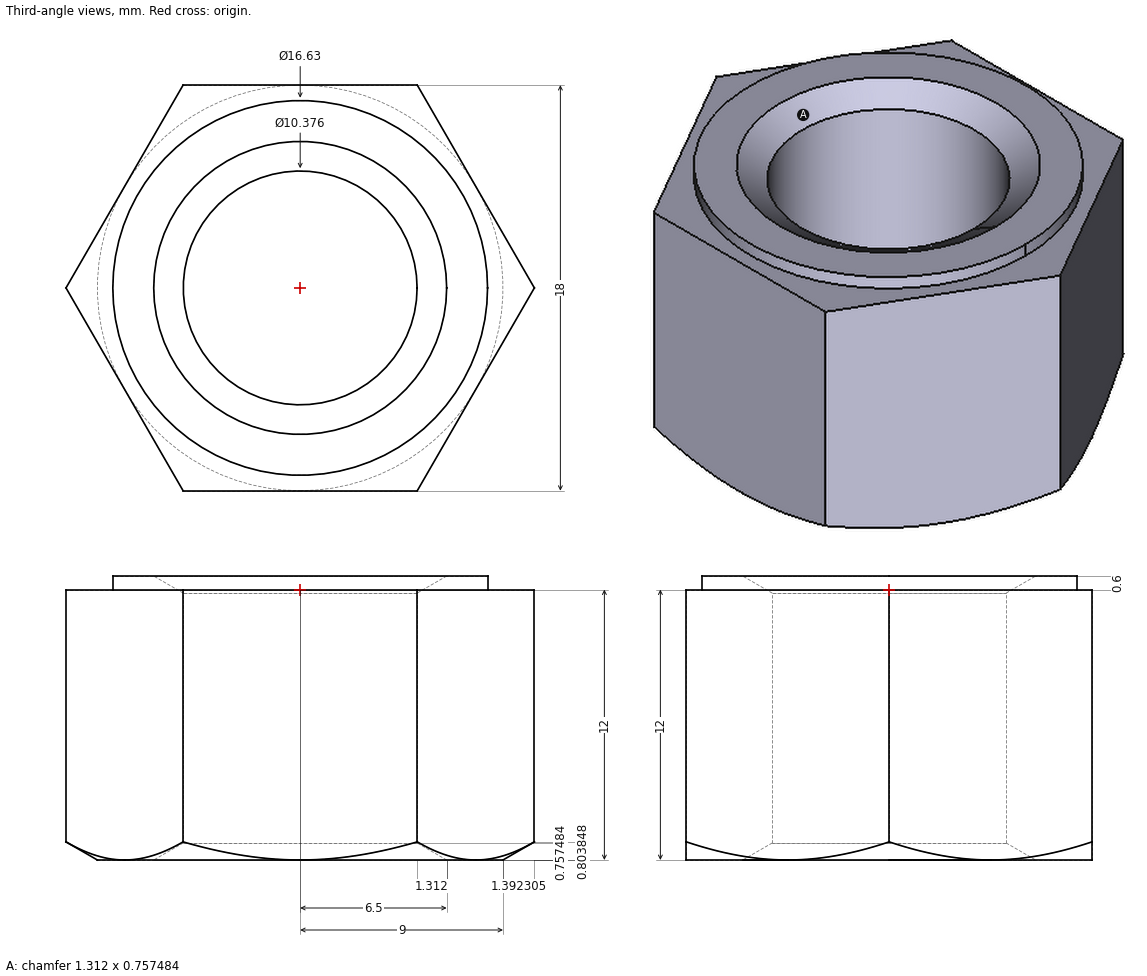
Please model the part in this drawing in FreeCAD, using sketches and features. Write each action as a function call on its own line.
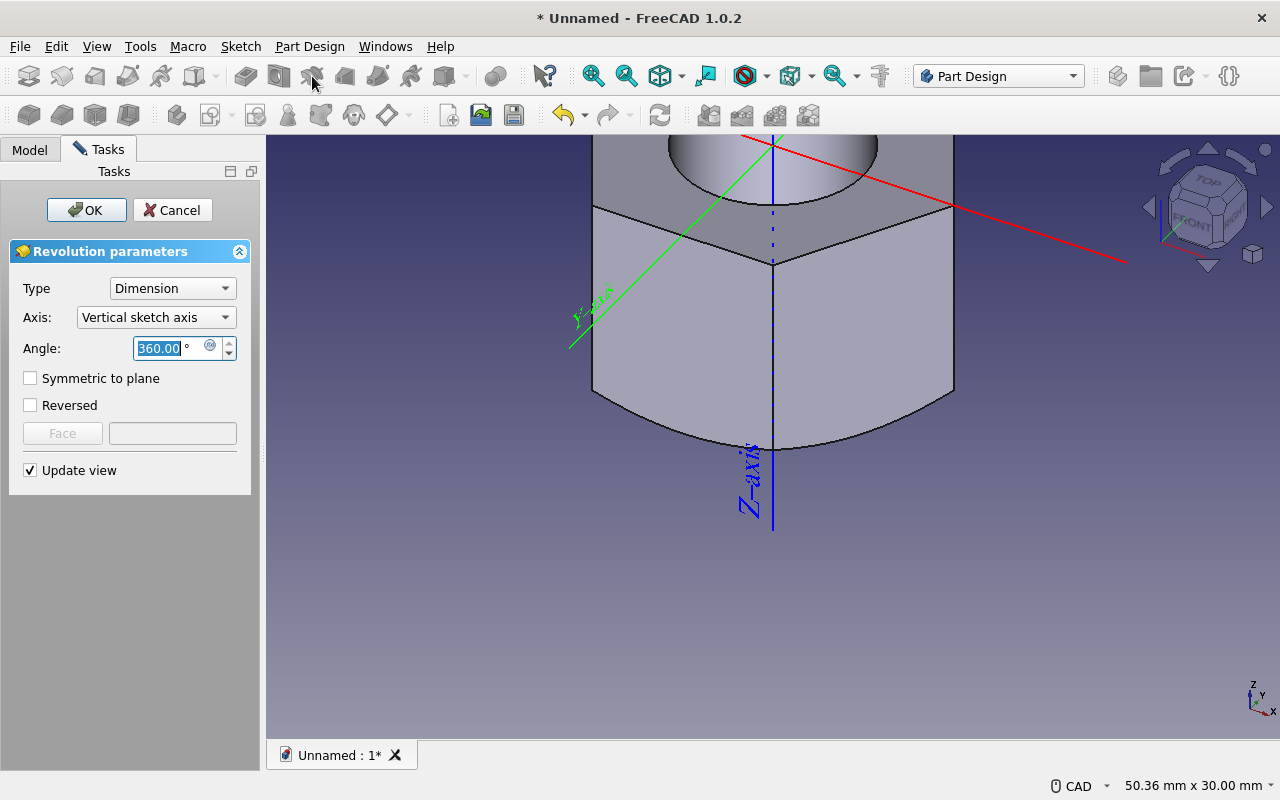
click(87, 210)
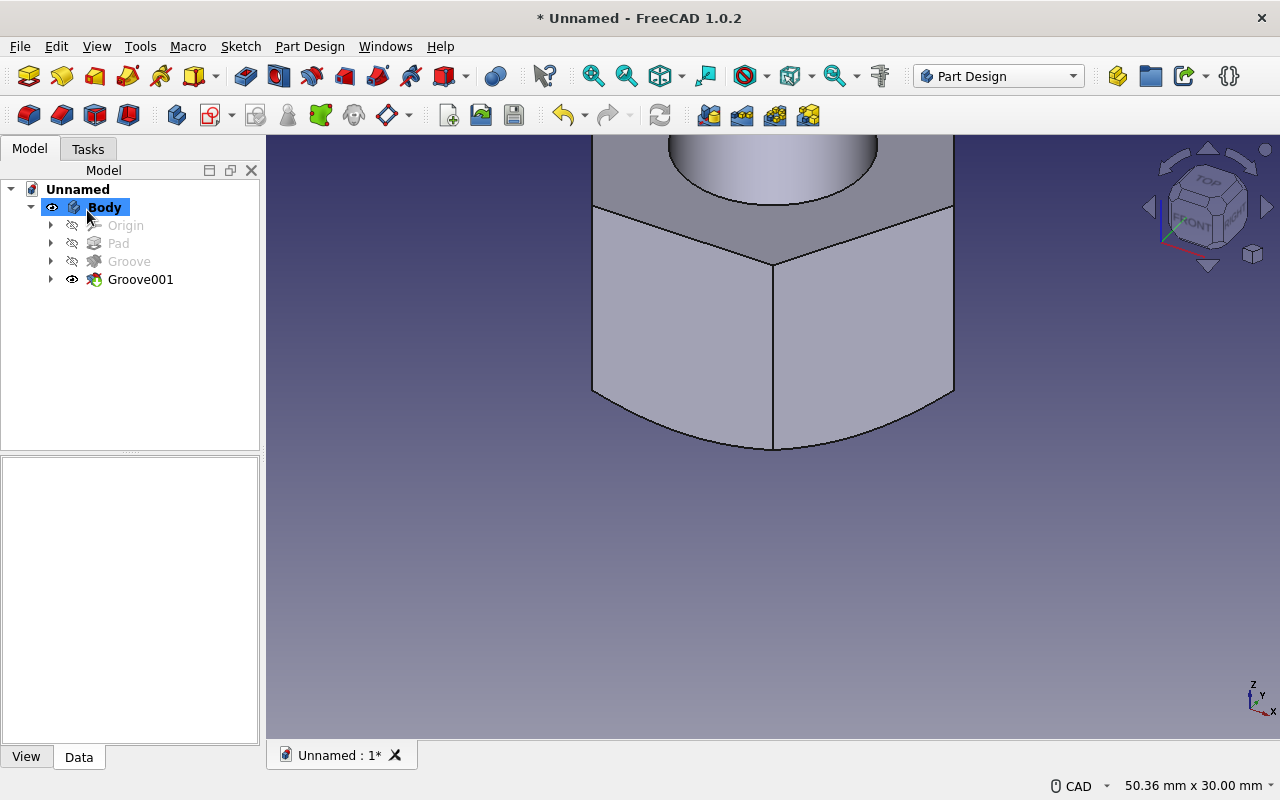
key(v)
key(f)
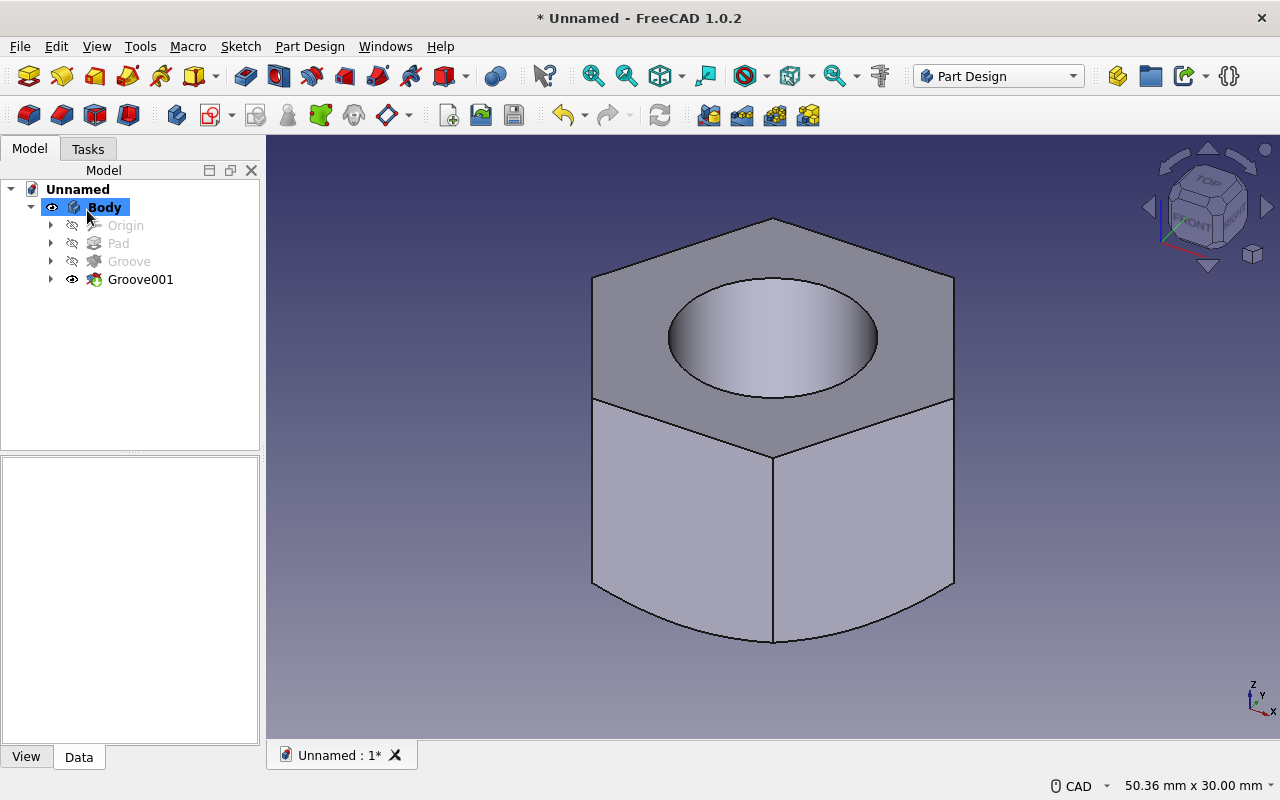
click(51, 225)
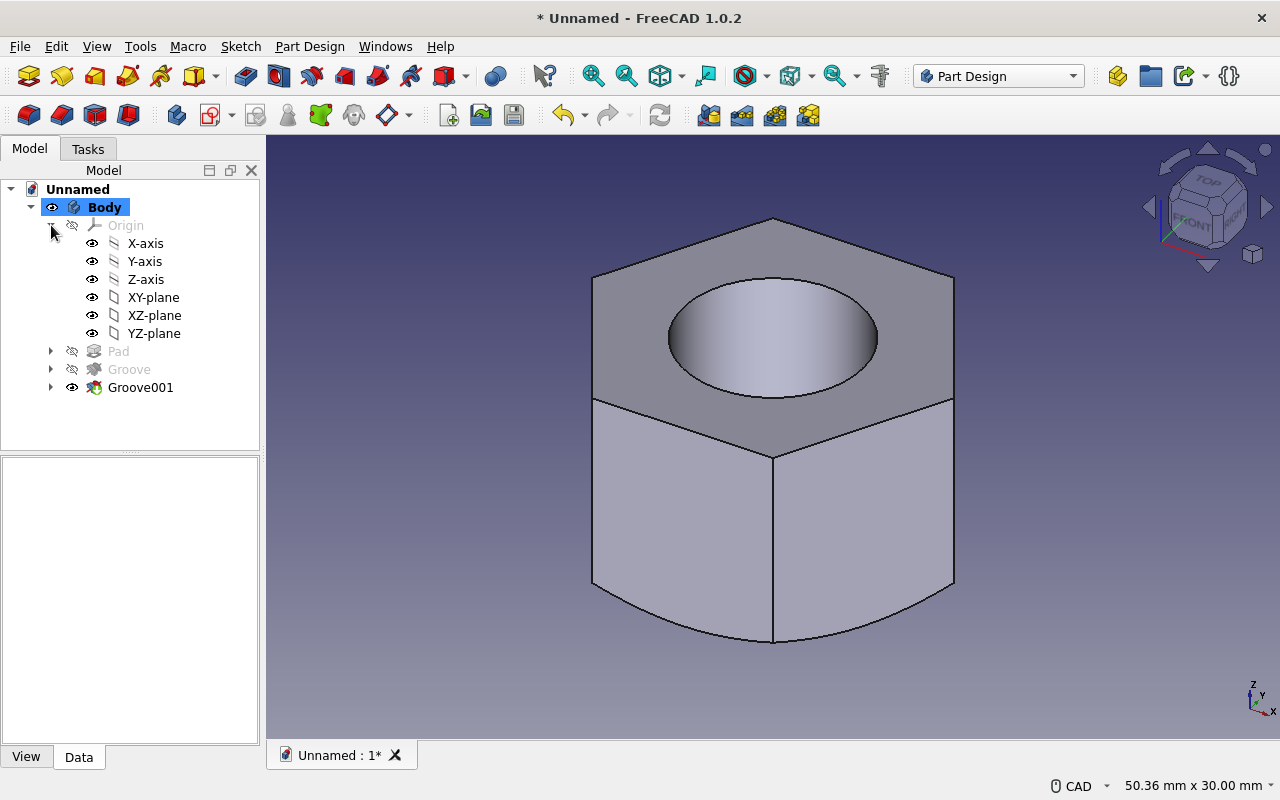
click(137, 297)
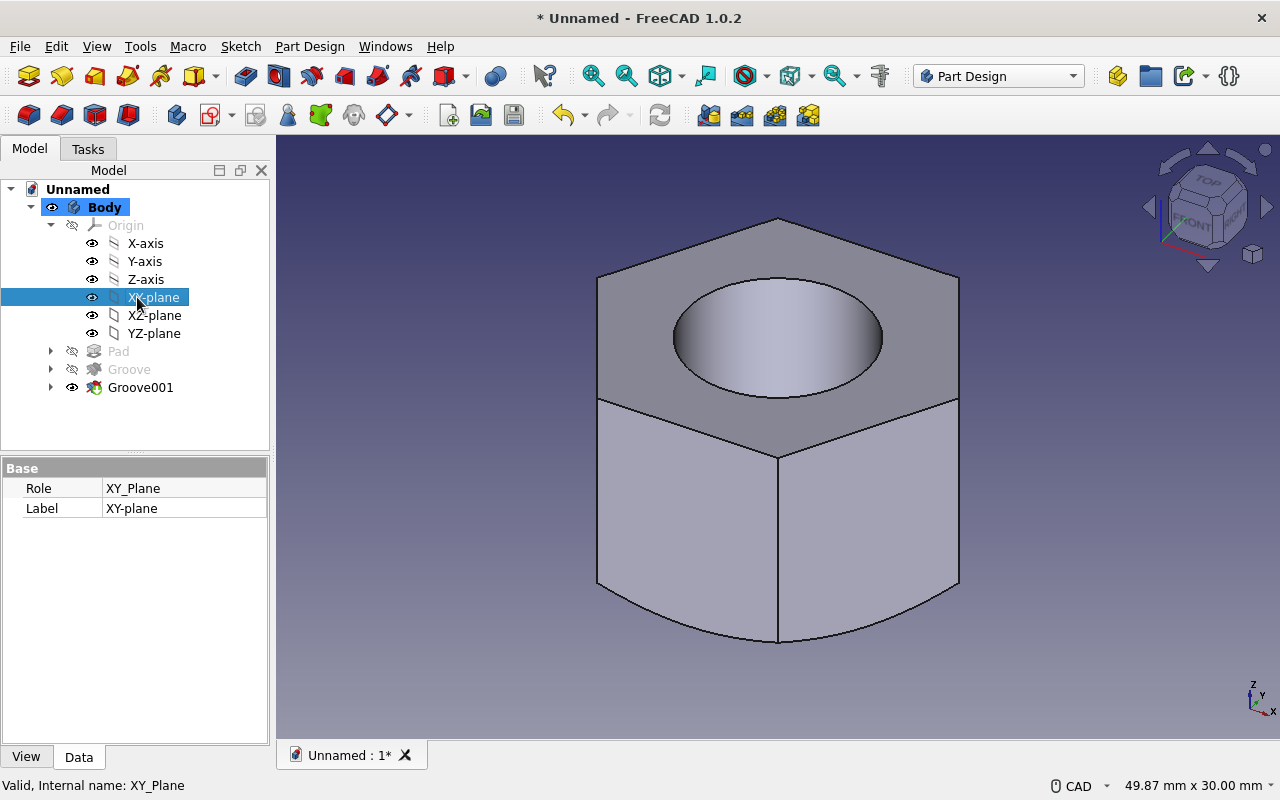
click(386, 116)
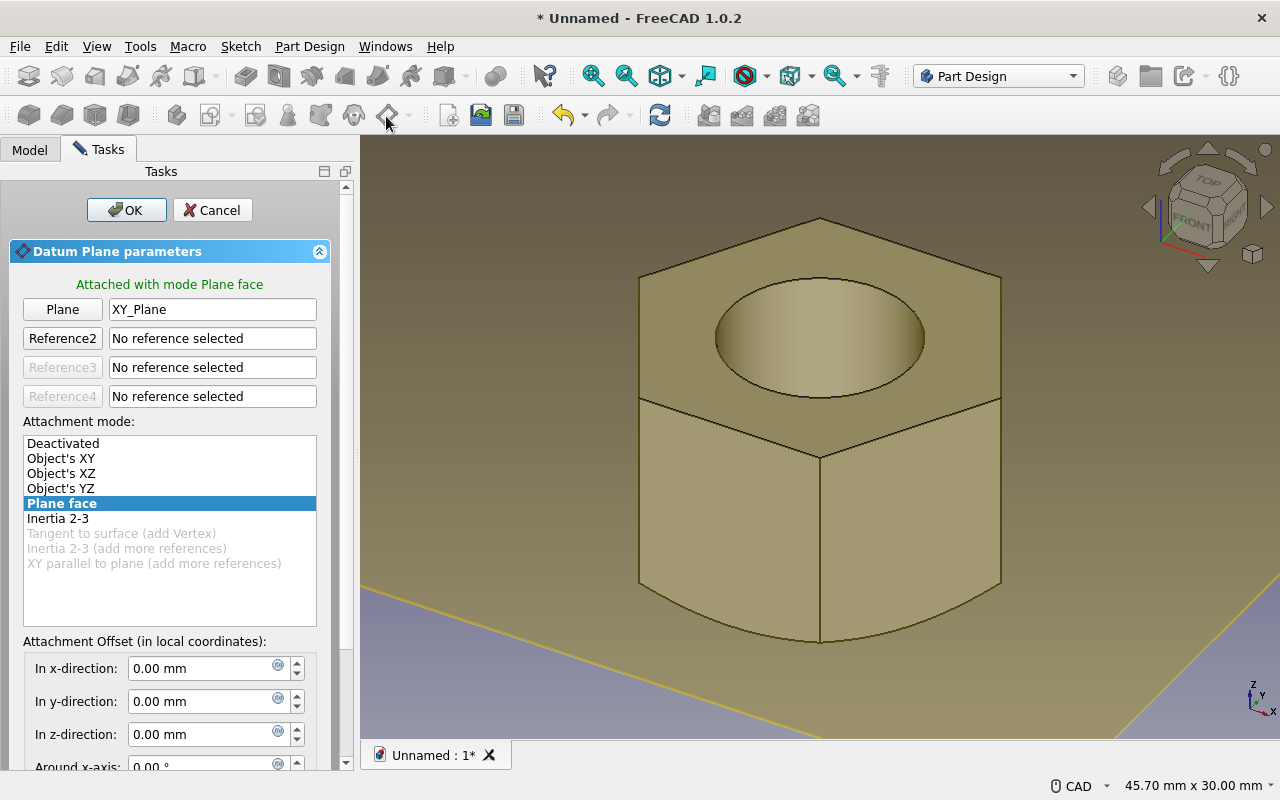
triple_click(210, 734)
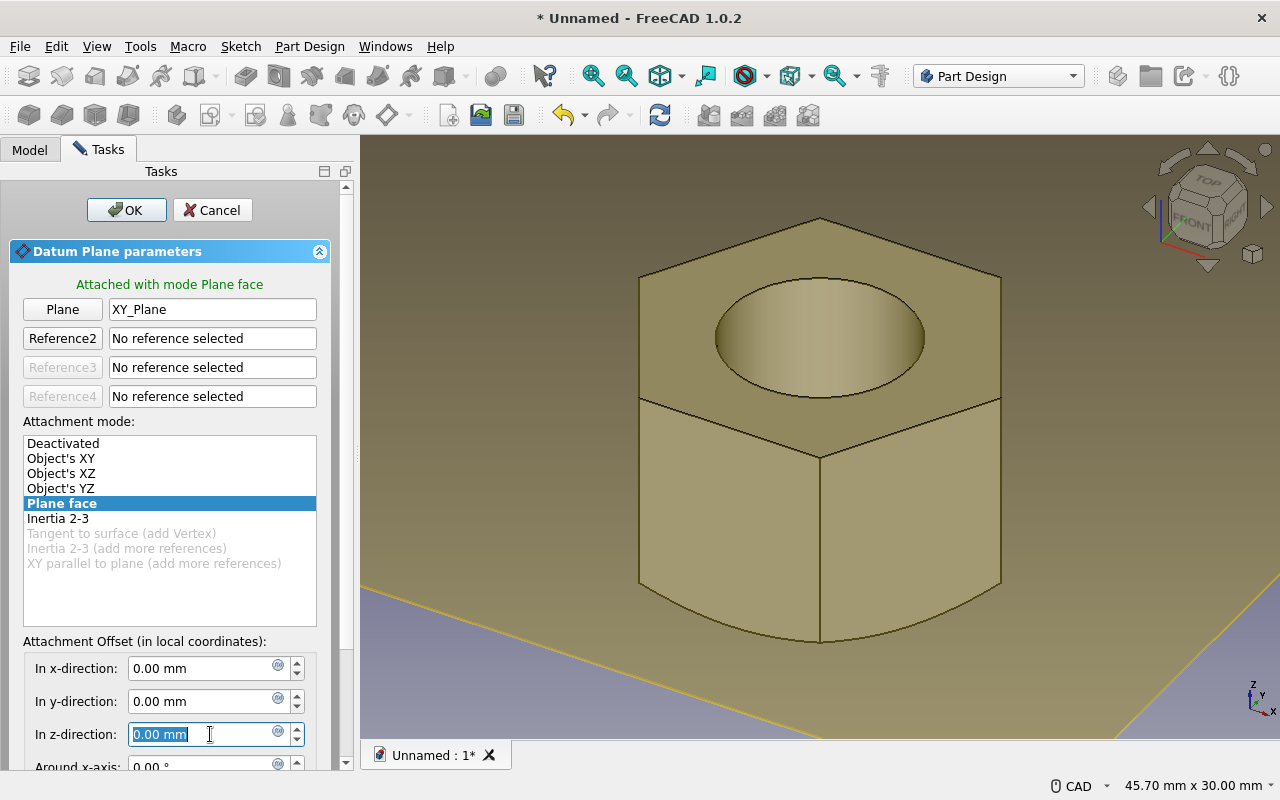
text(0.6)
key(Tab)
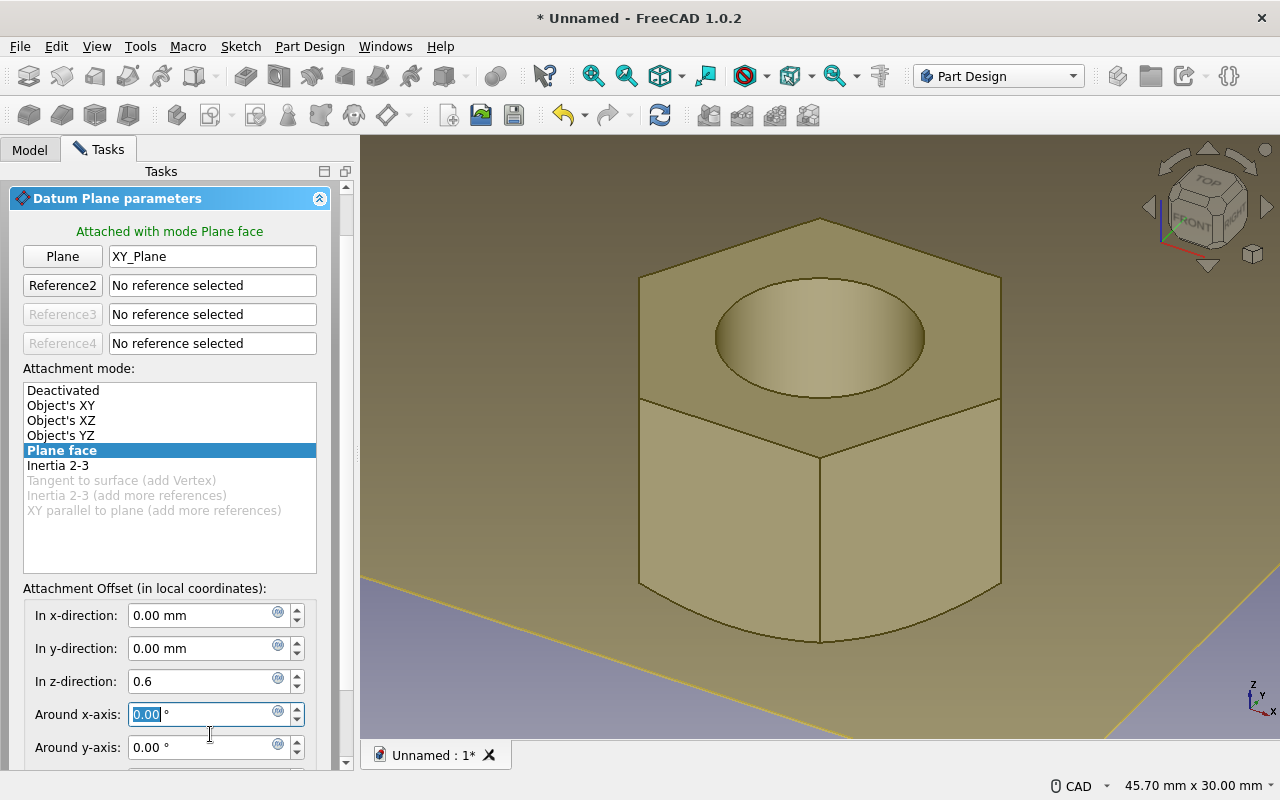
scroll(346, 476, up, 2)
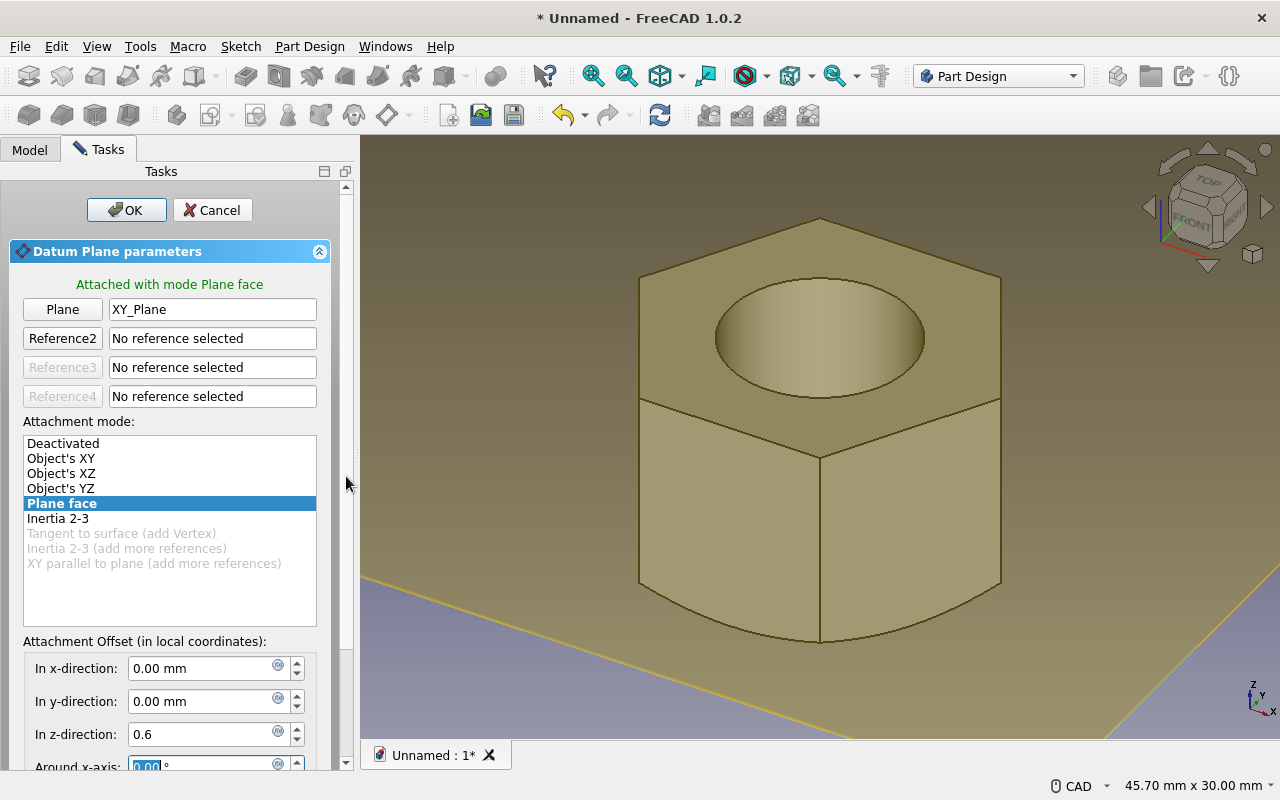
click(127, 210)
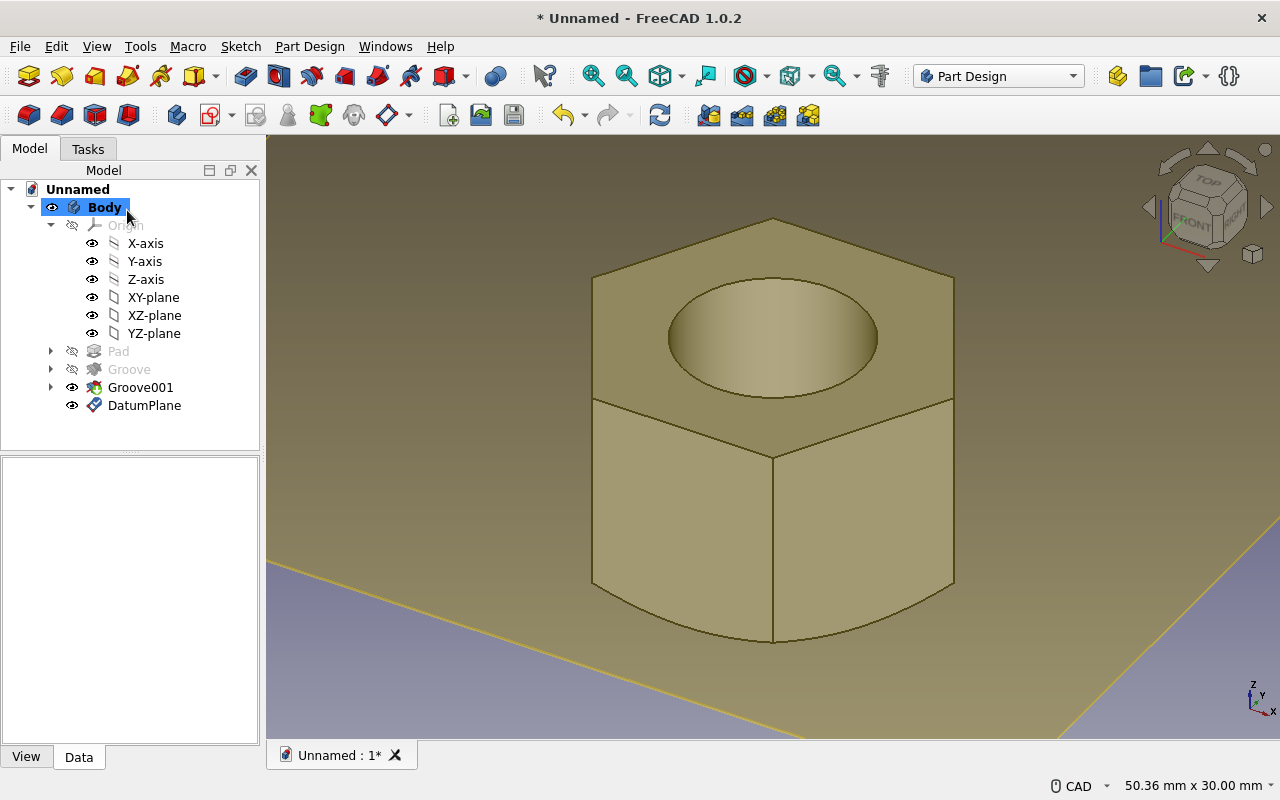
click(117, 405)